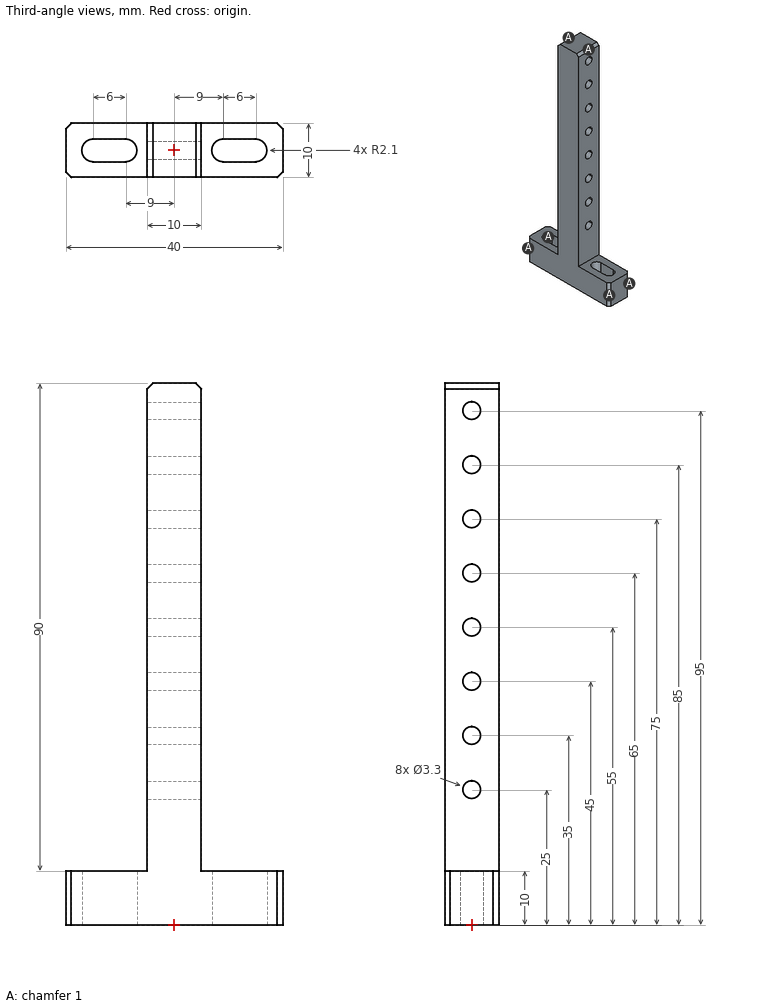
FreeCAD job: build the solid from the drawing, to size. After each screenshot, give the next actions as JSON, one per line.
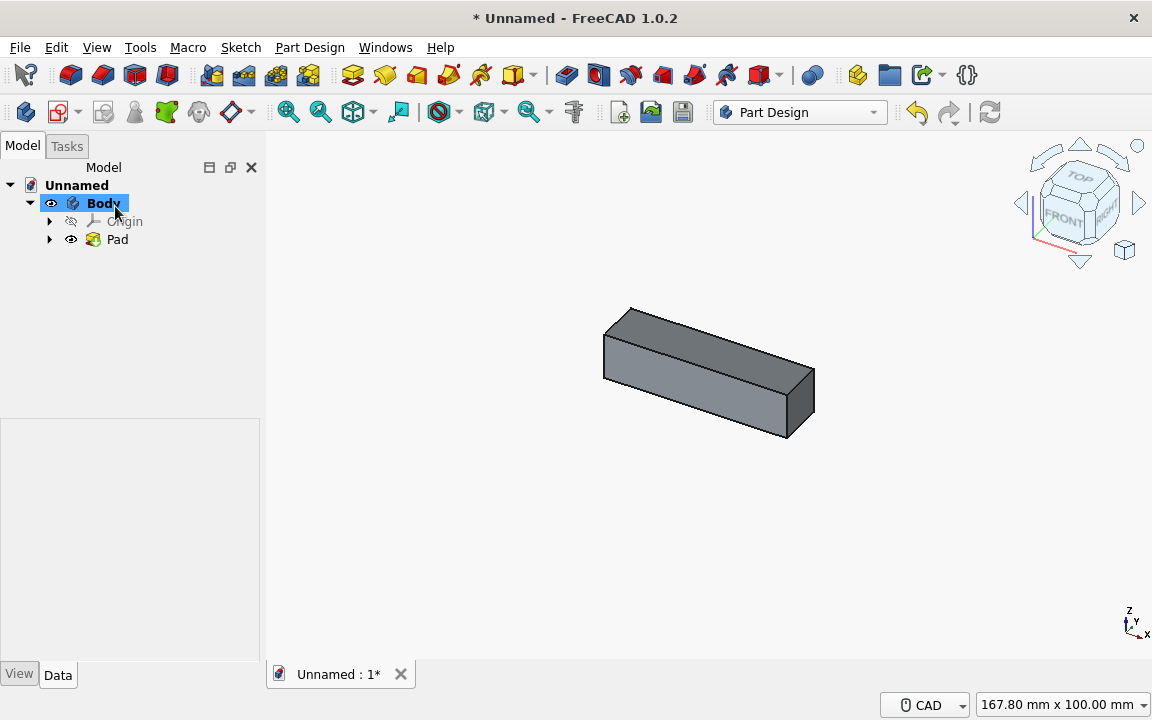
{"action": "left_click", "coordinate": [290, 112]}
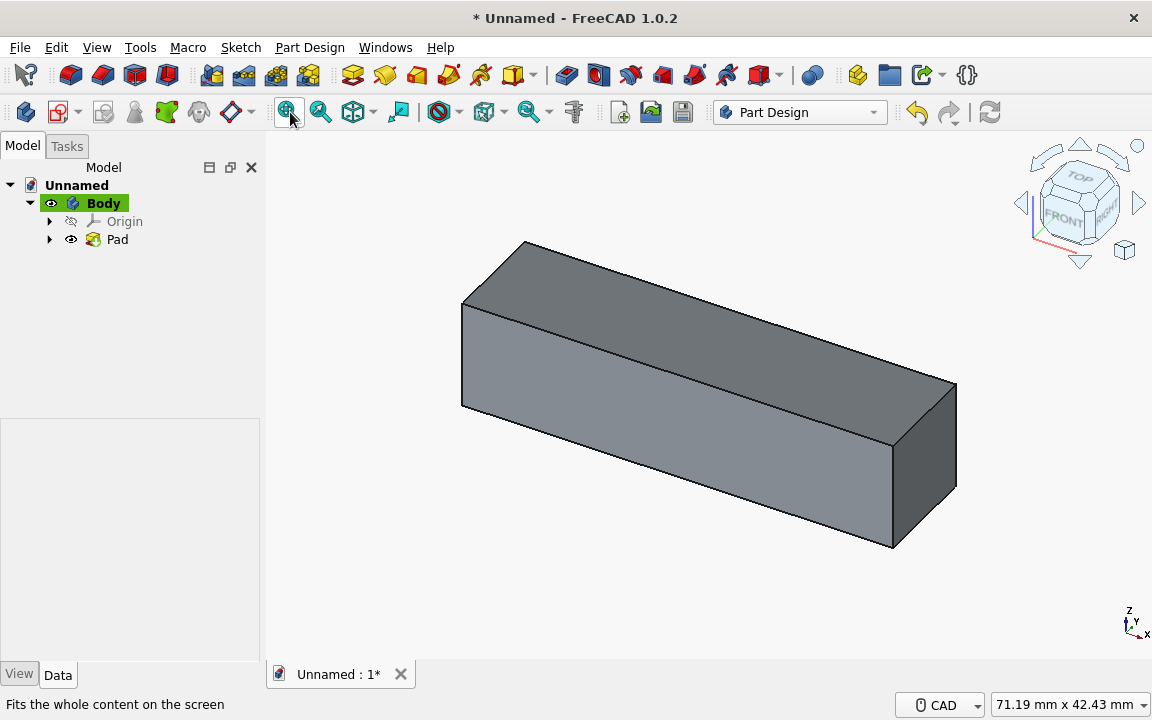
{"action": "left_click", "coordinate": [832, 384]}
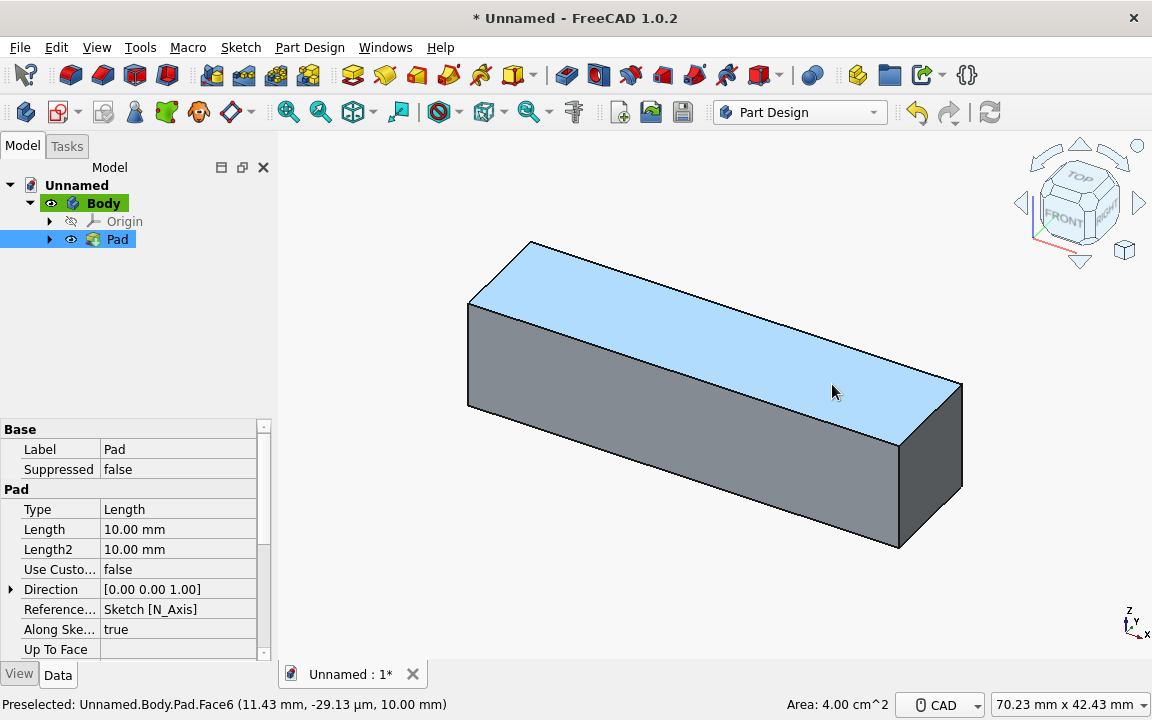
{"action": "left_click", "coordinate": [58, 112]}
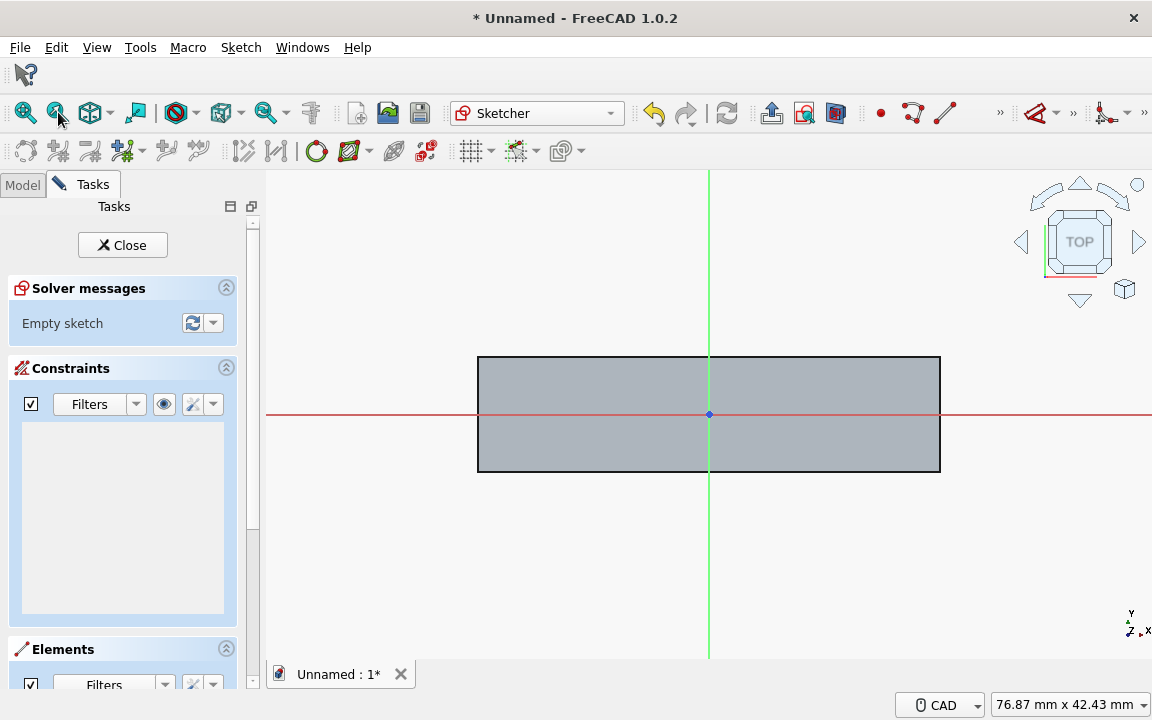
{"action": "scroll", "coordinate": [749, 415], "scroll_direction": "up", "scroll_amount": 5}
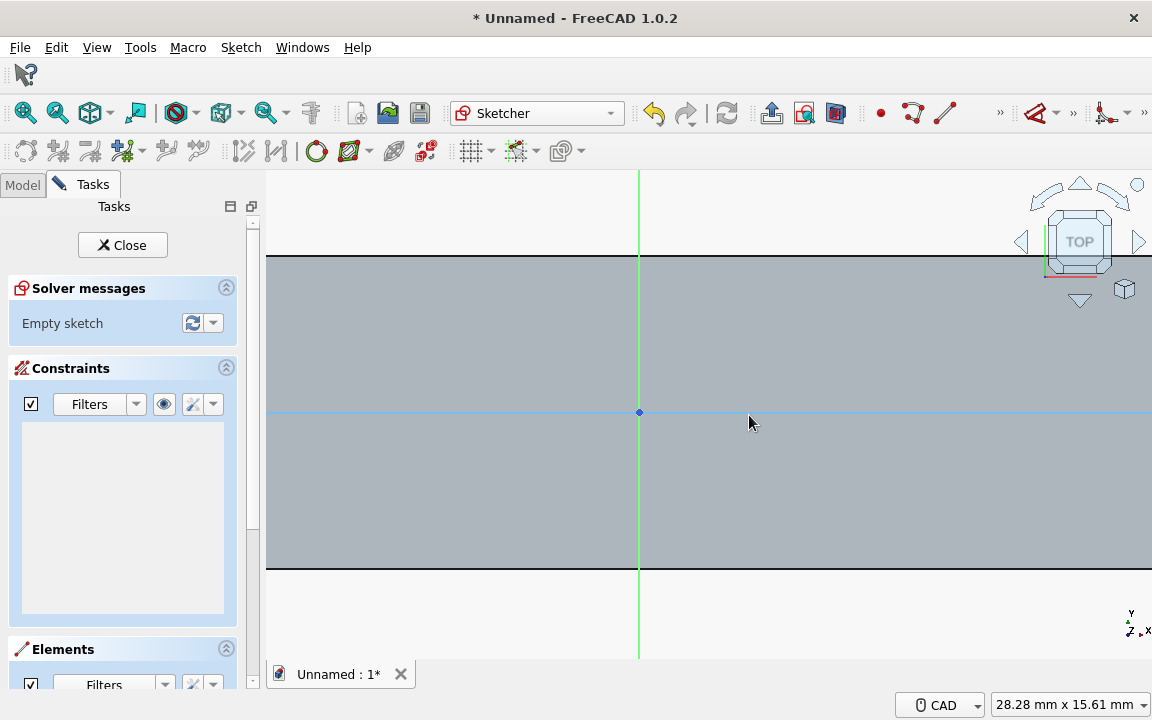
{"action": "key", "text": "g v"}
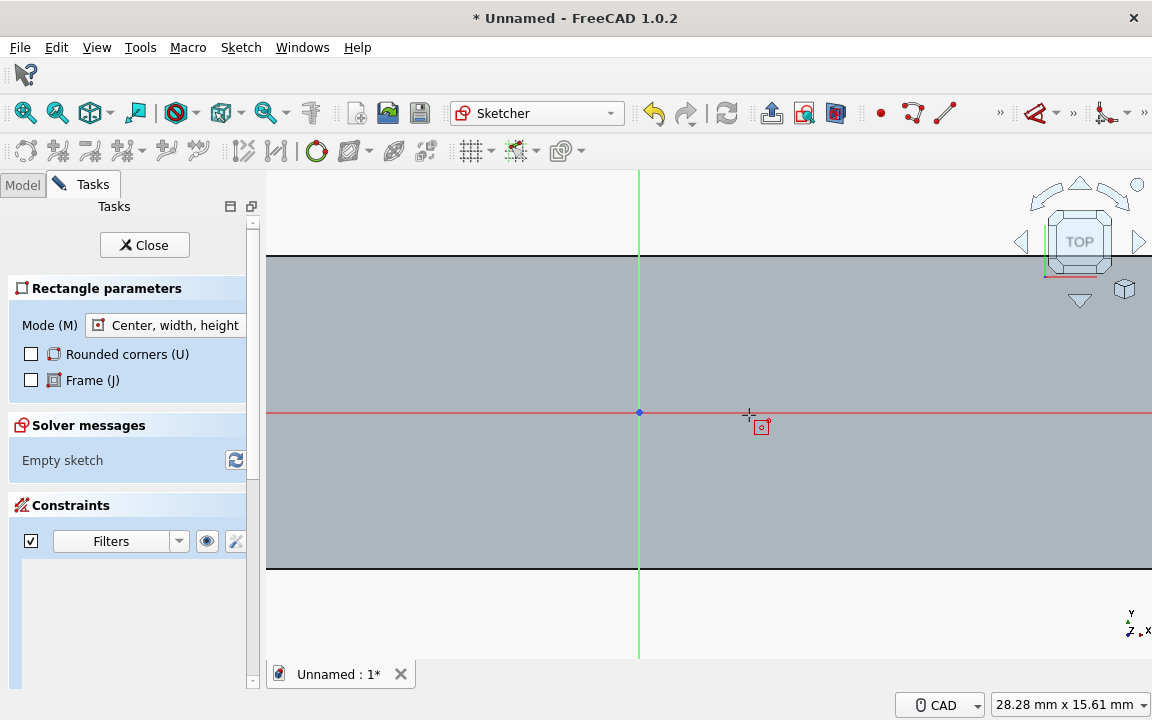
{"action": "left_click", "coordinate": [639, 413]}
{"action": "mouse_move", "coordinate": [796, 256]}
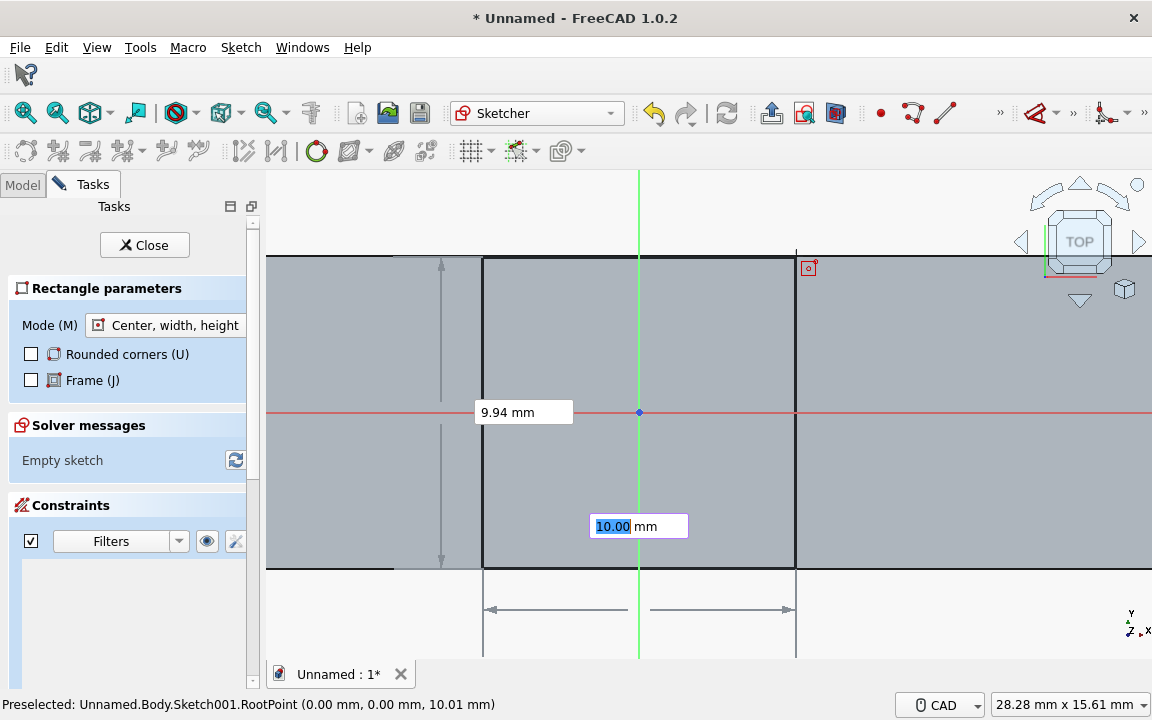
{"action": "type", "text": "10"}
{"action": "key", "text": "Tab"}
{"action": "type", "text": "10"}
{"action": "key", "text": "Return"}
{"action": "key", "text": "Escape"}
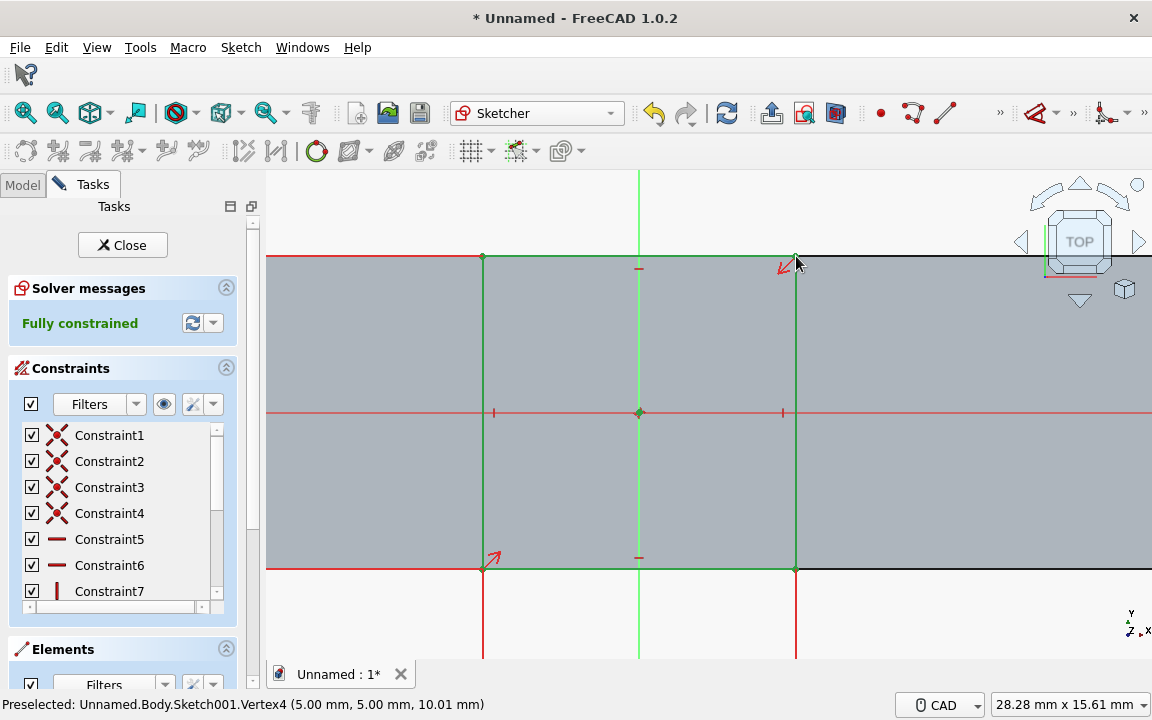
{"action": "left_click", "coordinate": [123, 245]}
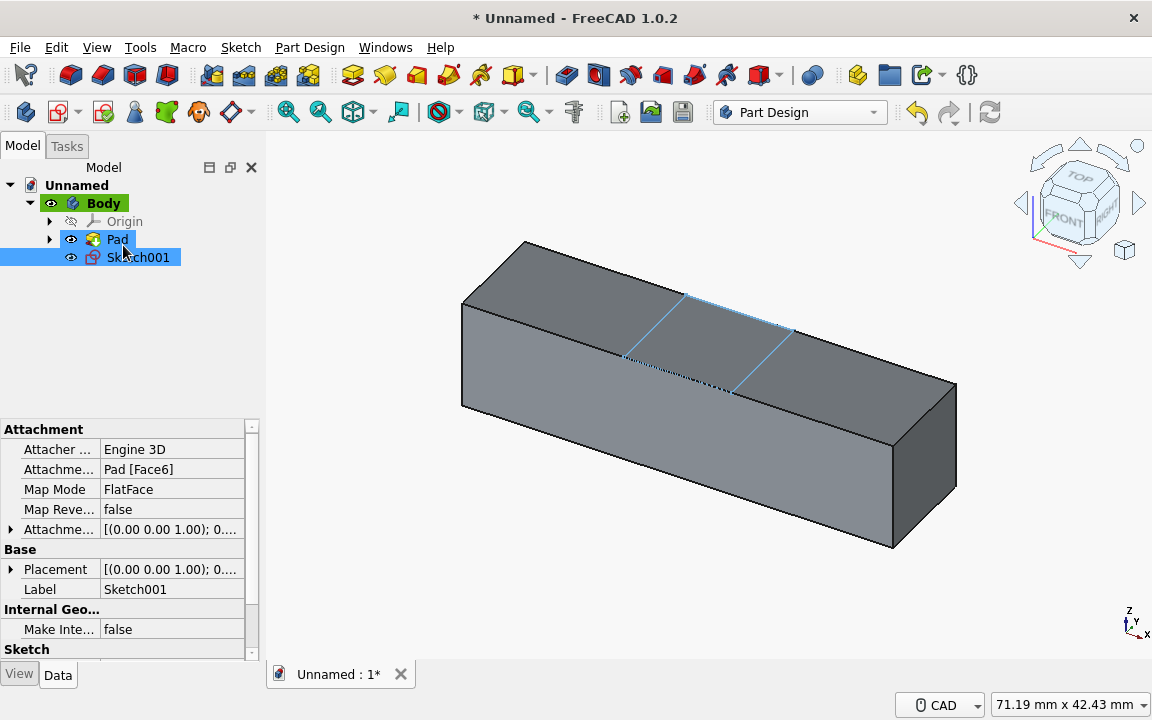
{"action": "left_click", "coordinate": [354, 76]}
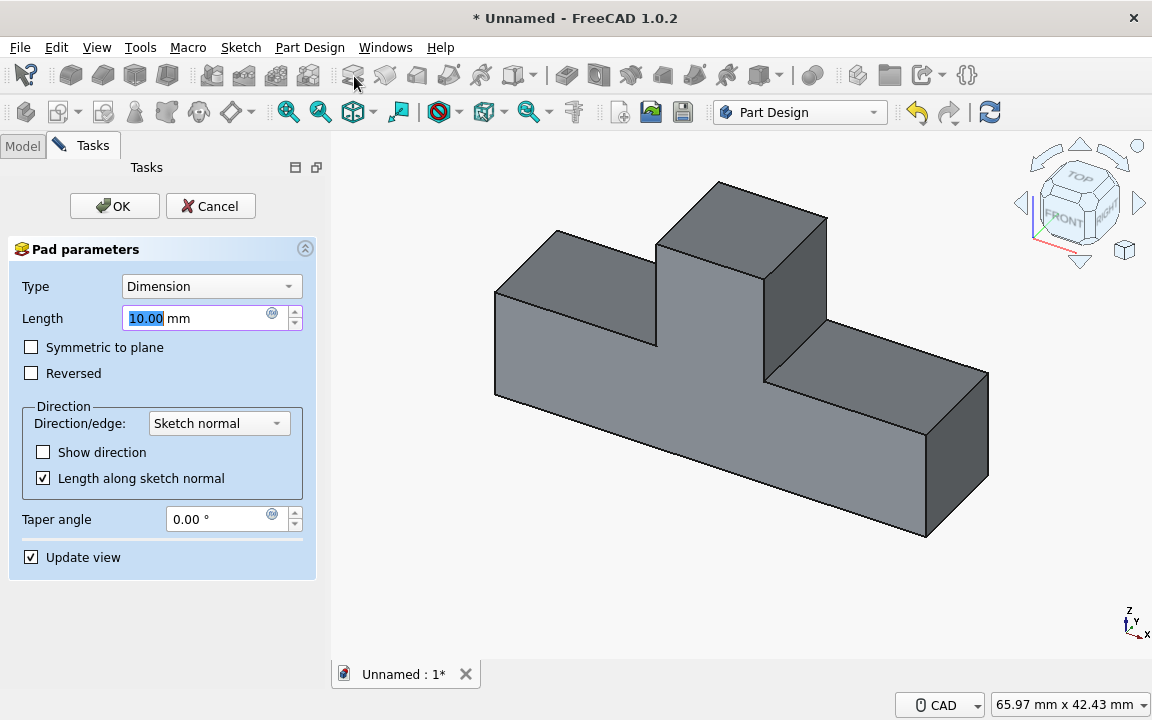
{"action": "type", "text": "90"}
{"action": "key", "text": "Tab"}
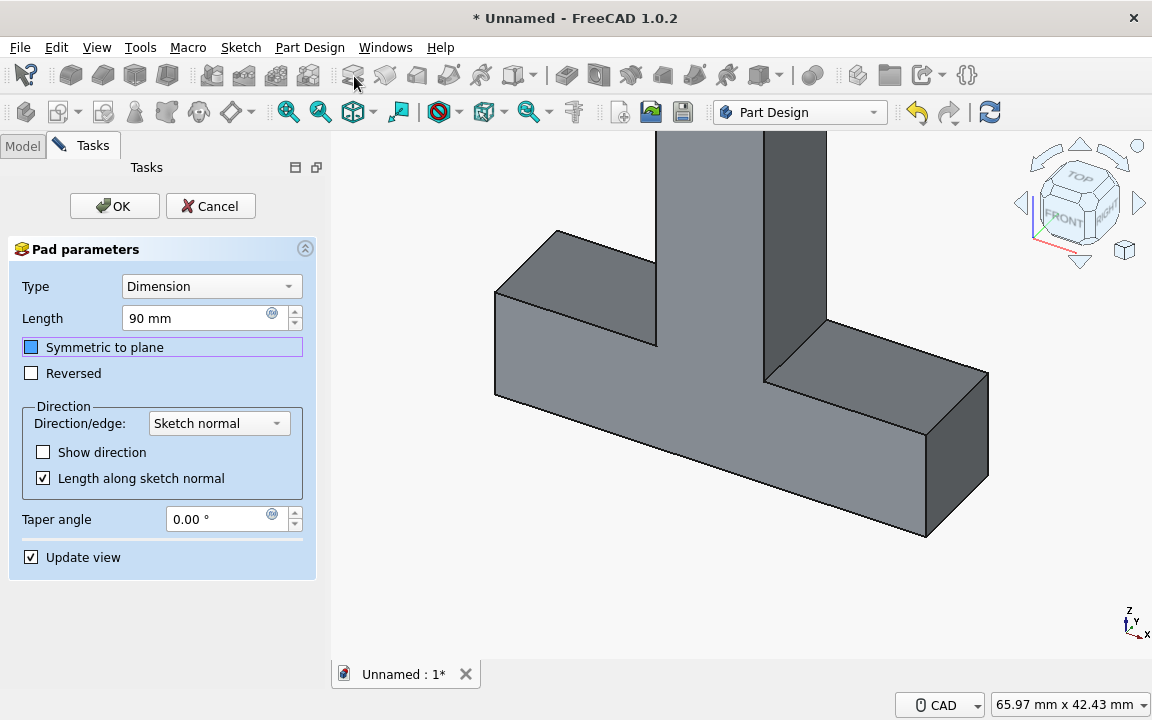
{"action": "left_click", "coordinate": [115, 206]}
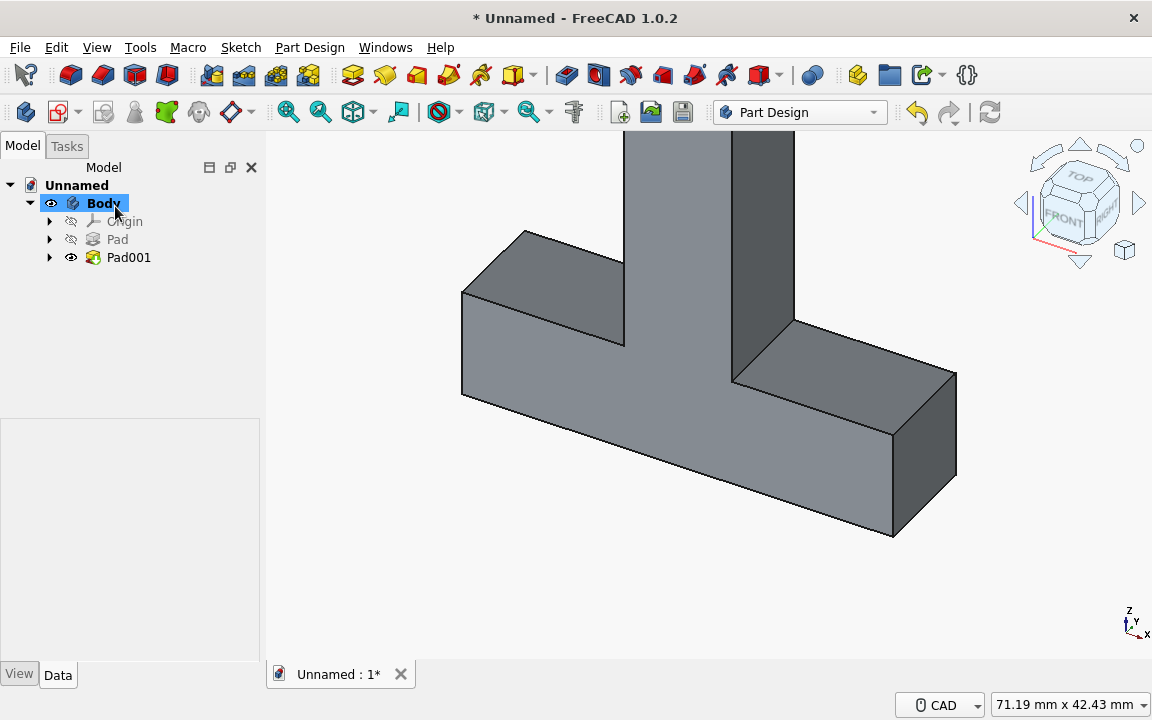
{"action": "left_click", "coordinate": [290, 112]}